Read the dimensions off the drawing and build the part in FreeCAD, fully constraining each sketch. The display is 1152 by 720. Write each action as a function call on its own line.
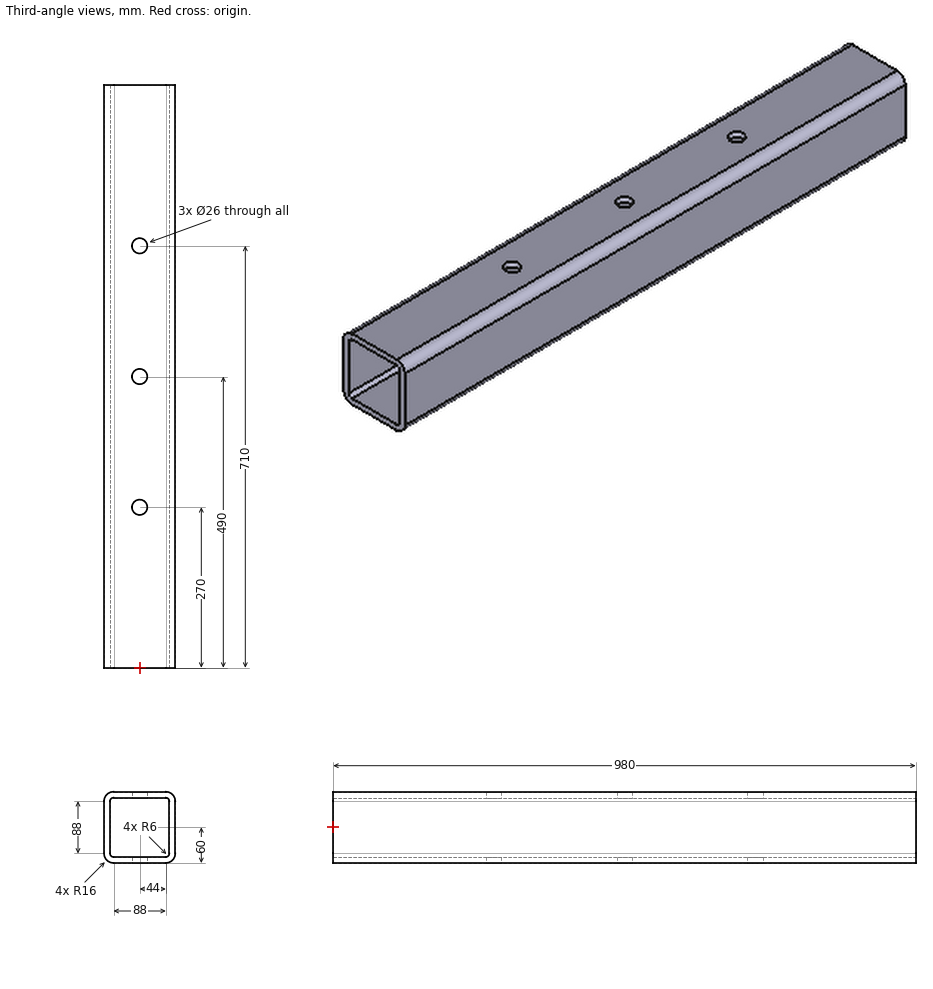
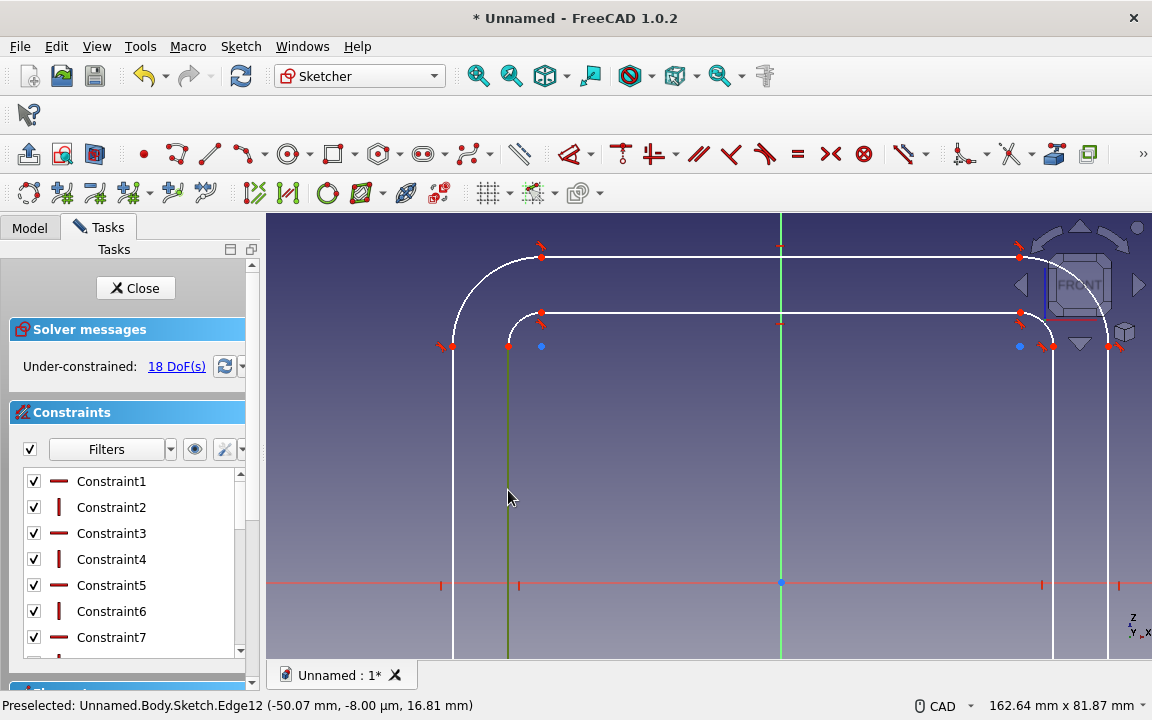
click(527, 316)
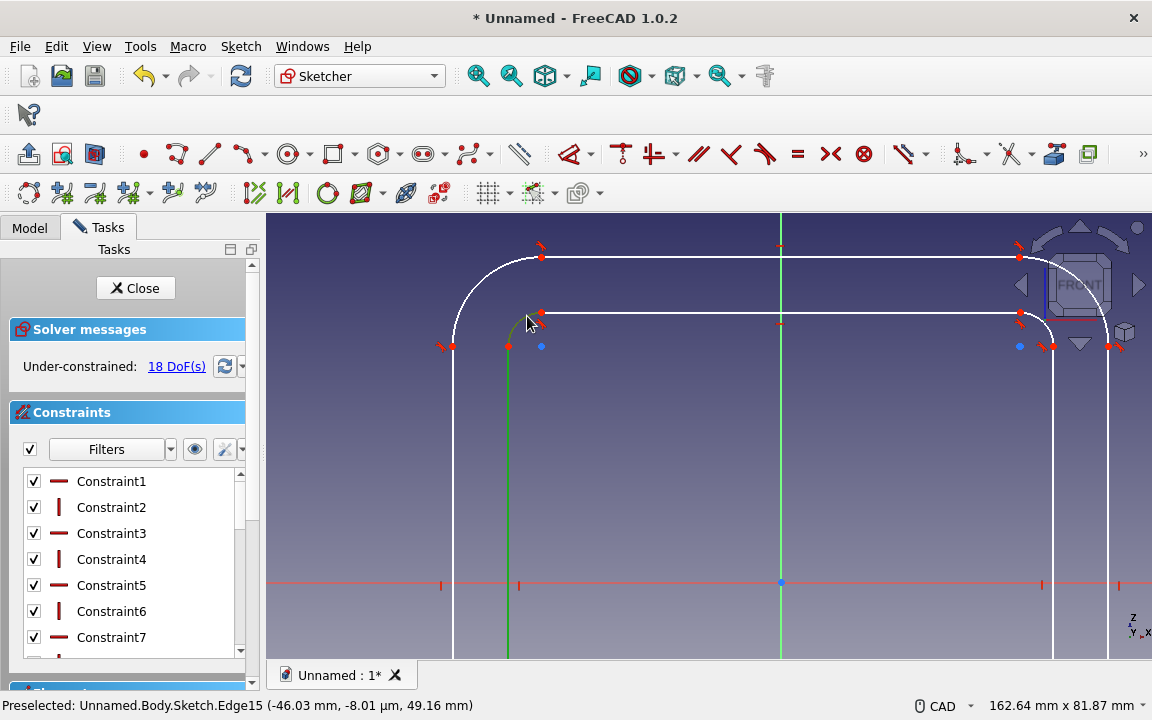
click(765, 154)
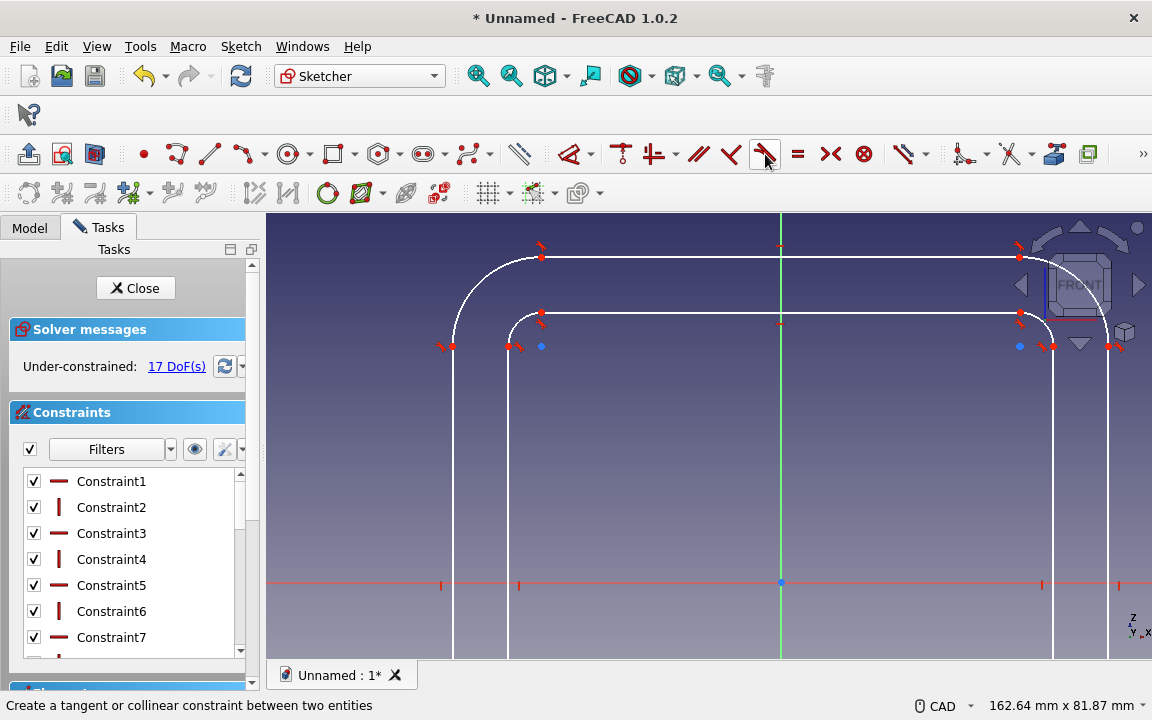
click(508, 490)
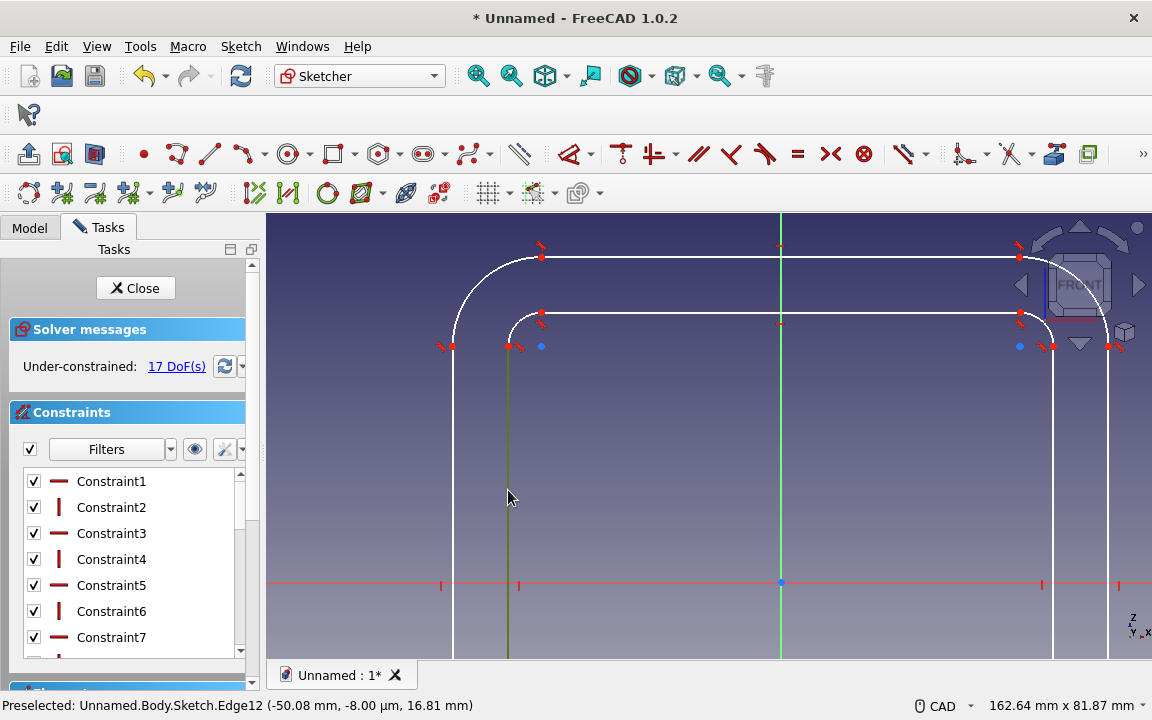
scroll(526, 316, down, 4)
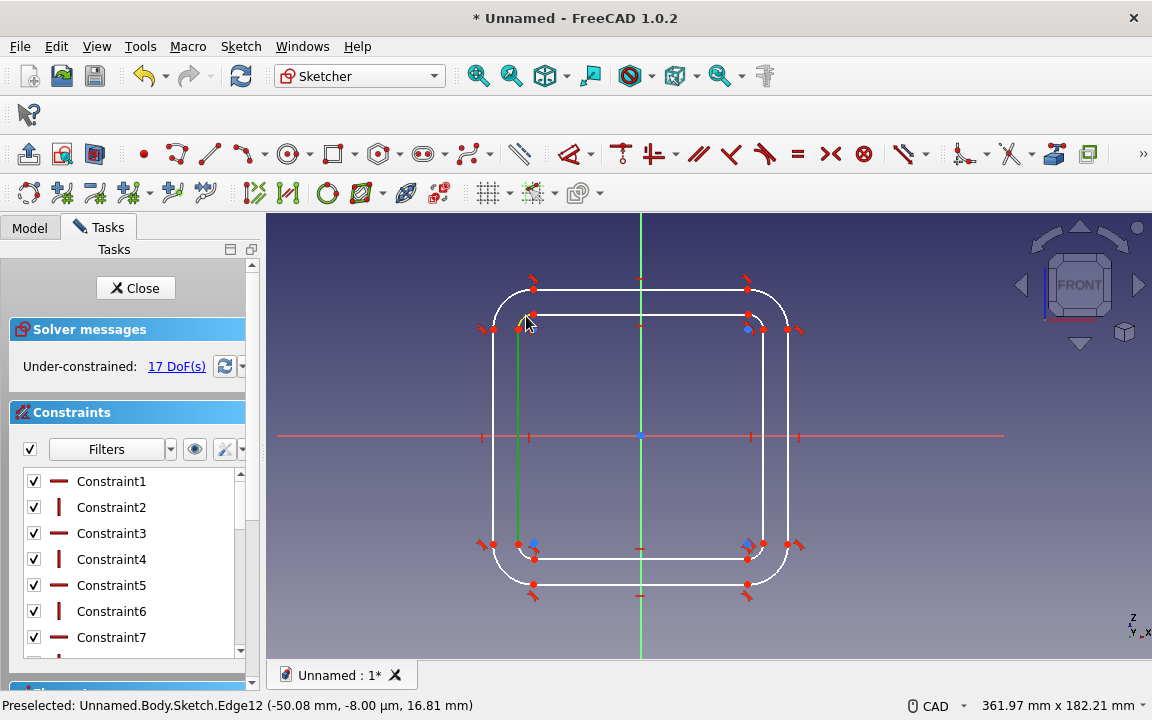
scroll(521, 551, up, 4)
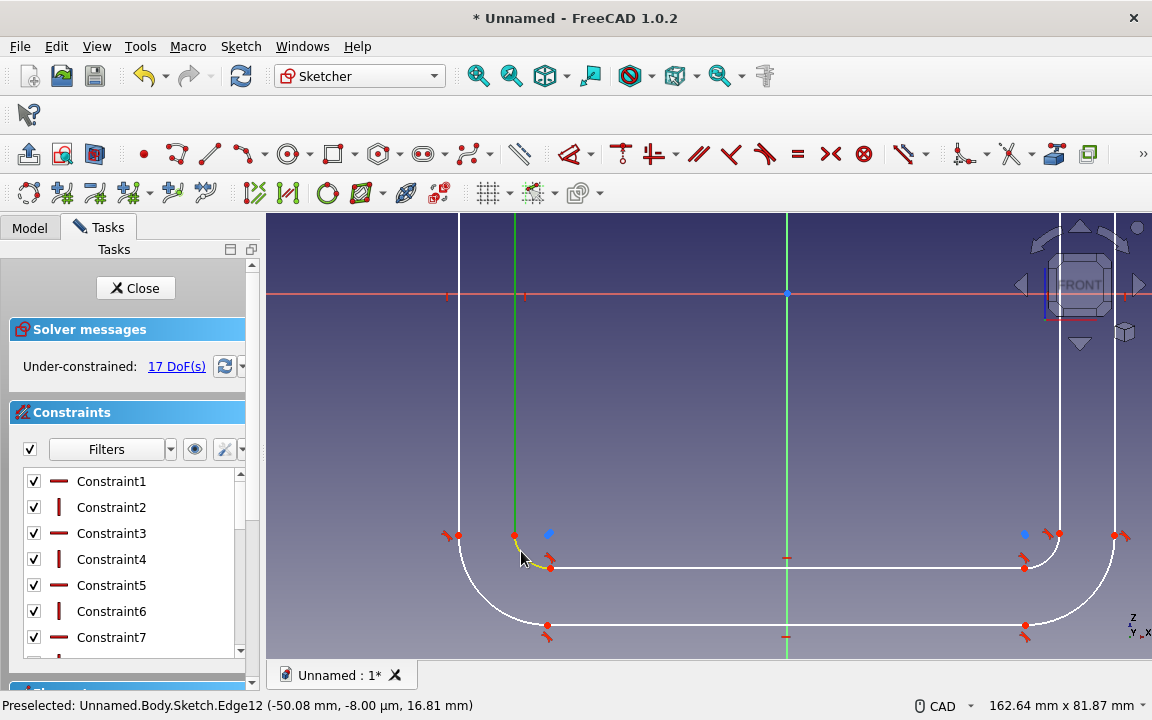
click(520, 551)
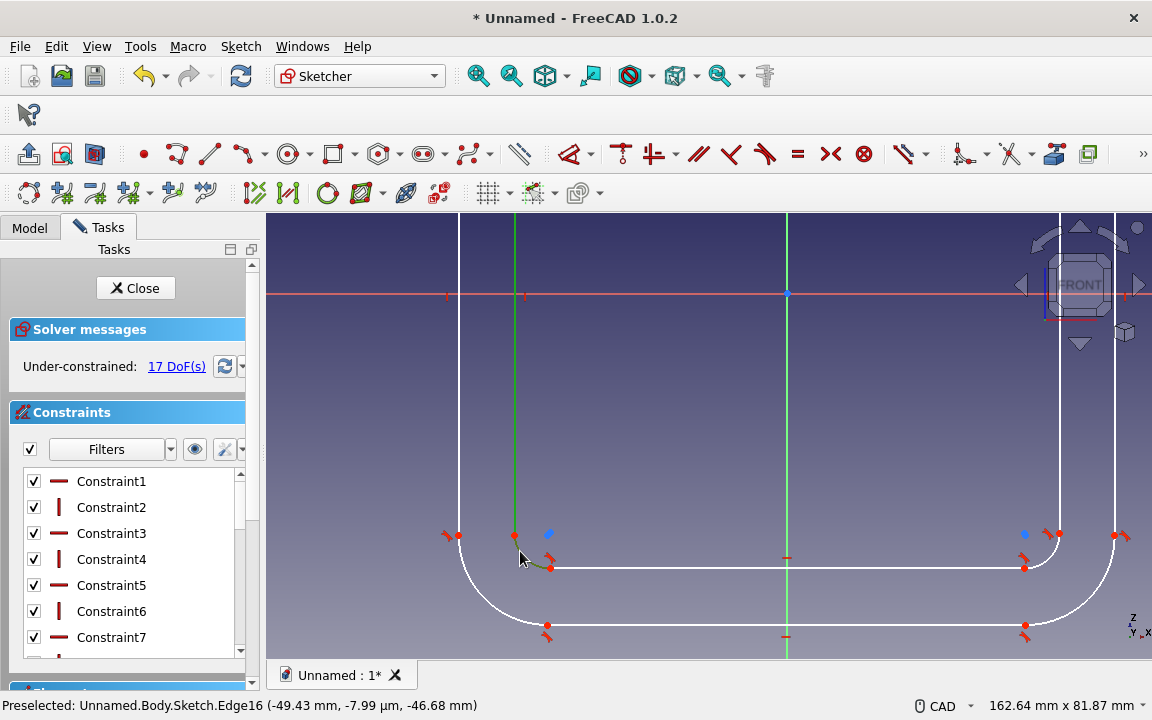
click(765, 154)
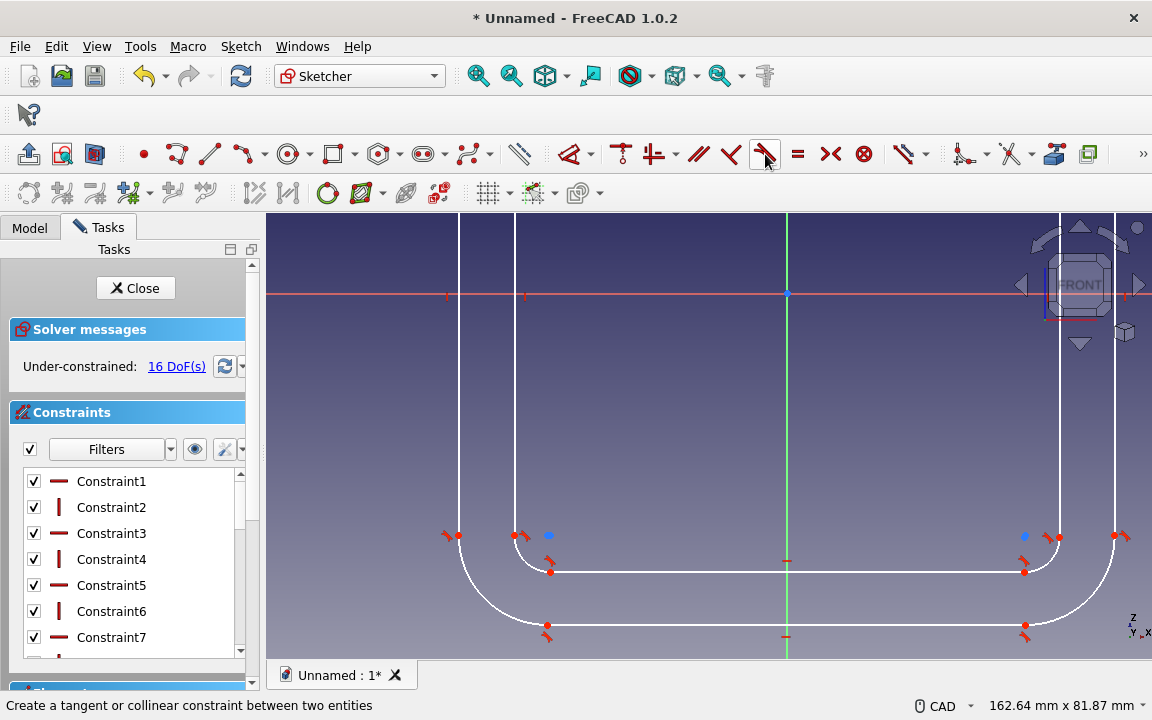
scroll(521, 552, down, 4)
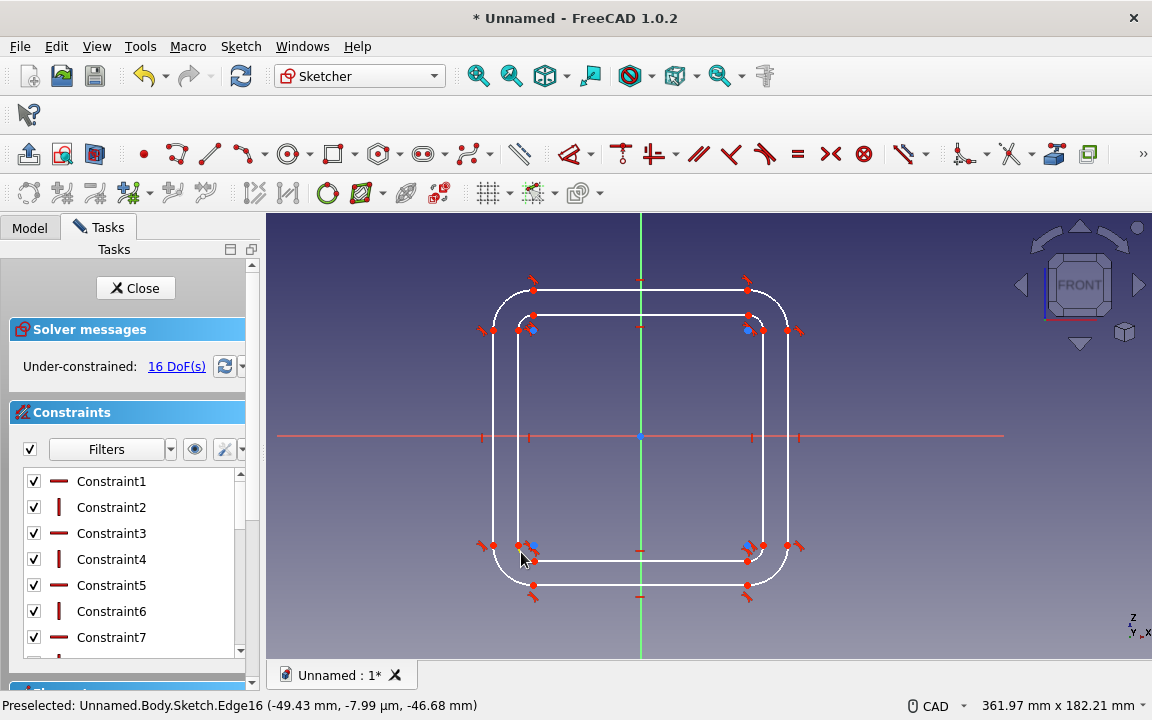
click(766, 581)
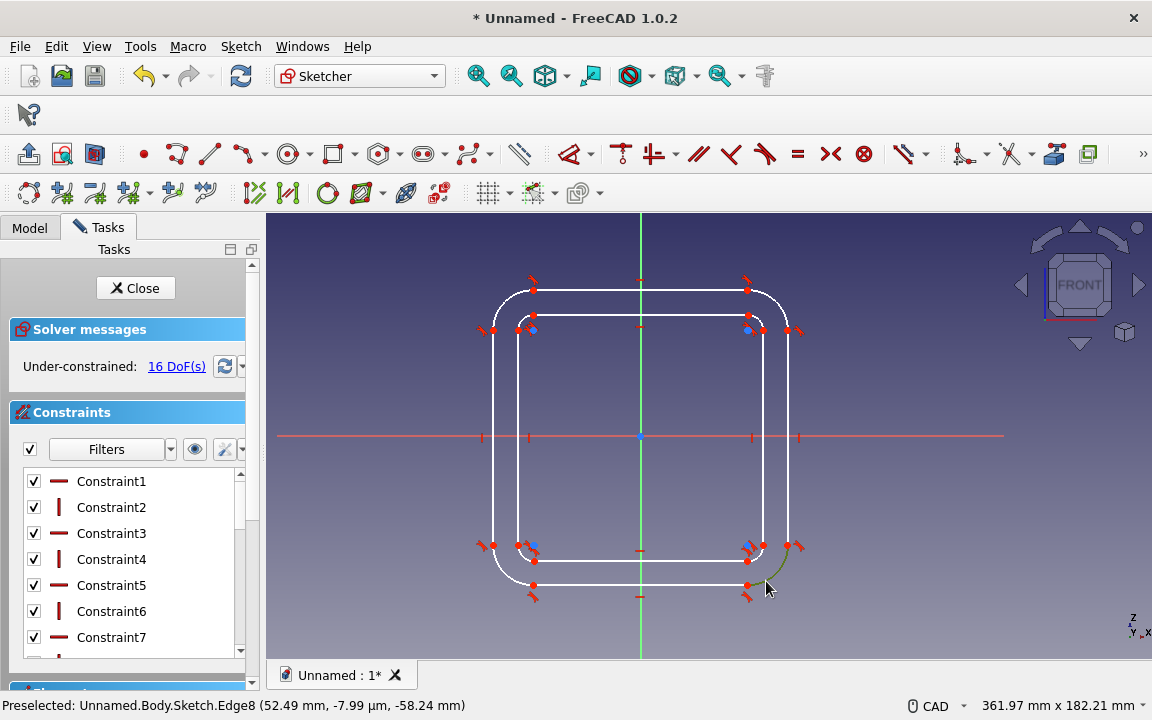
click(759, 557)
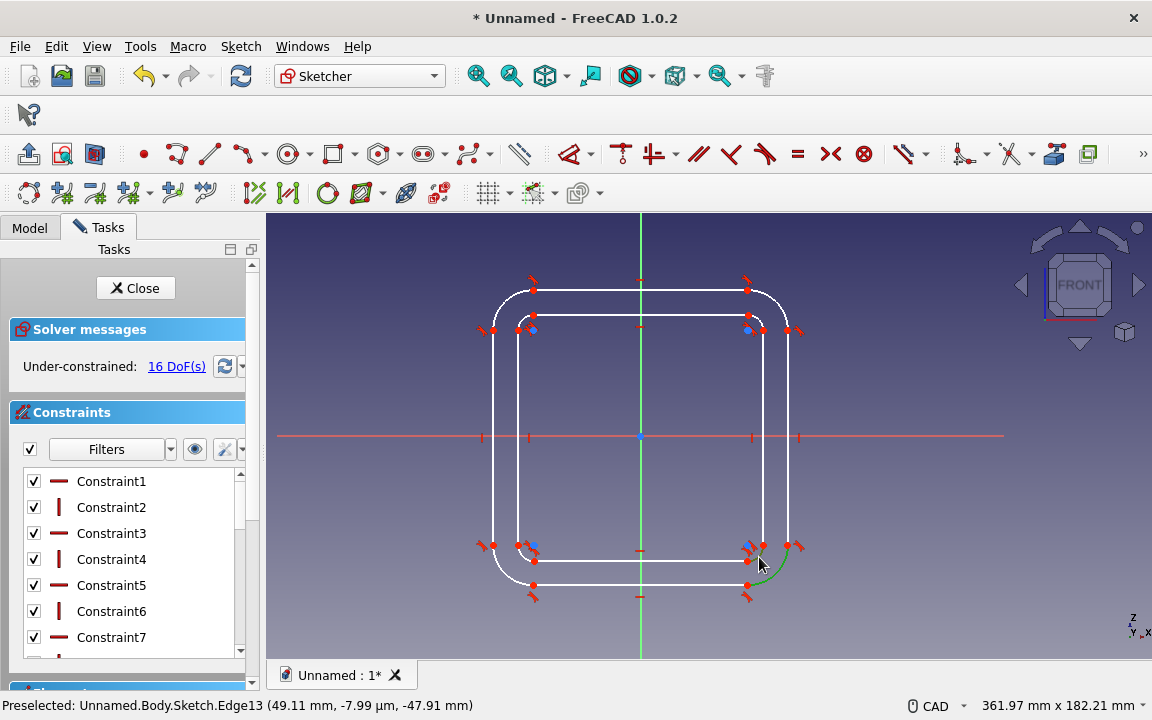
click(621, 154)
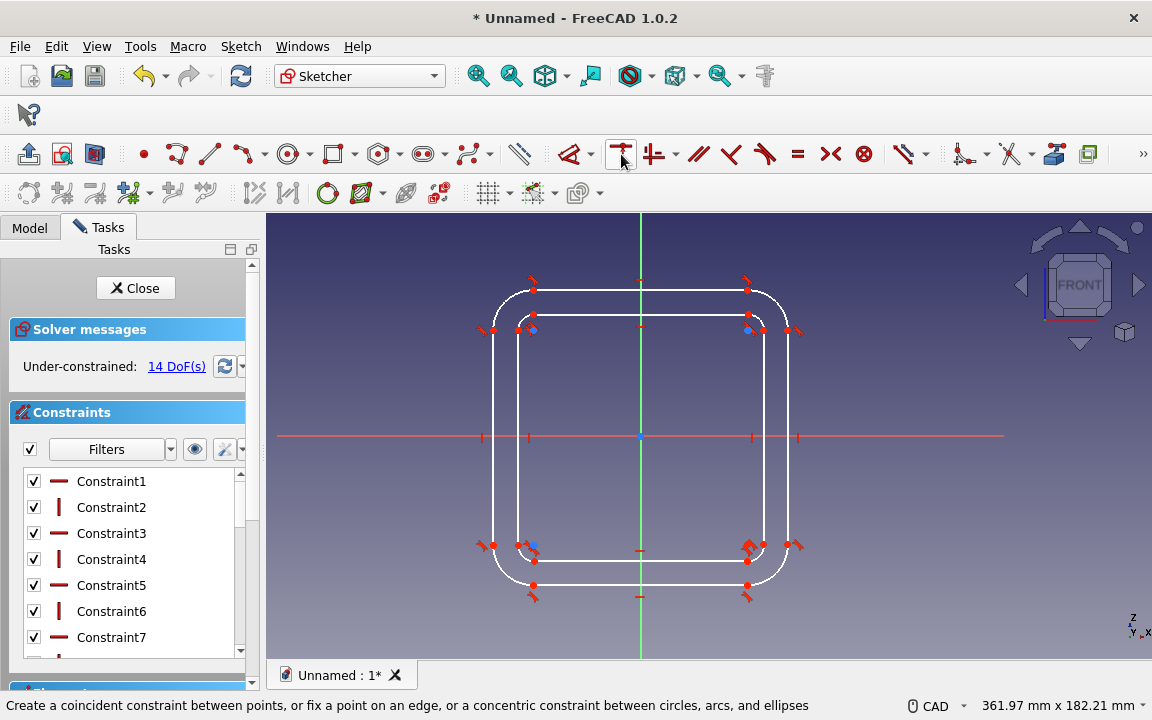
click(783, 312)